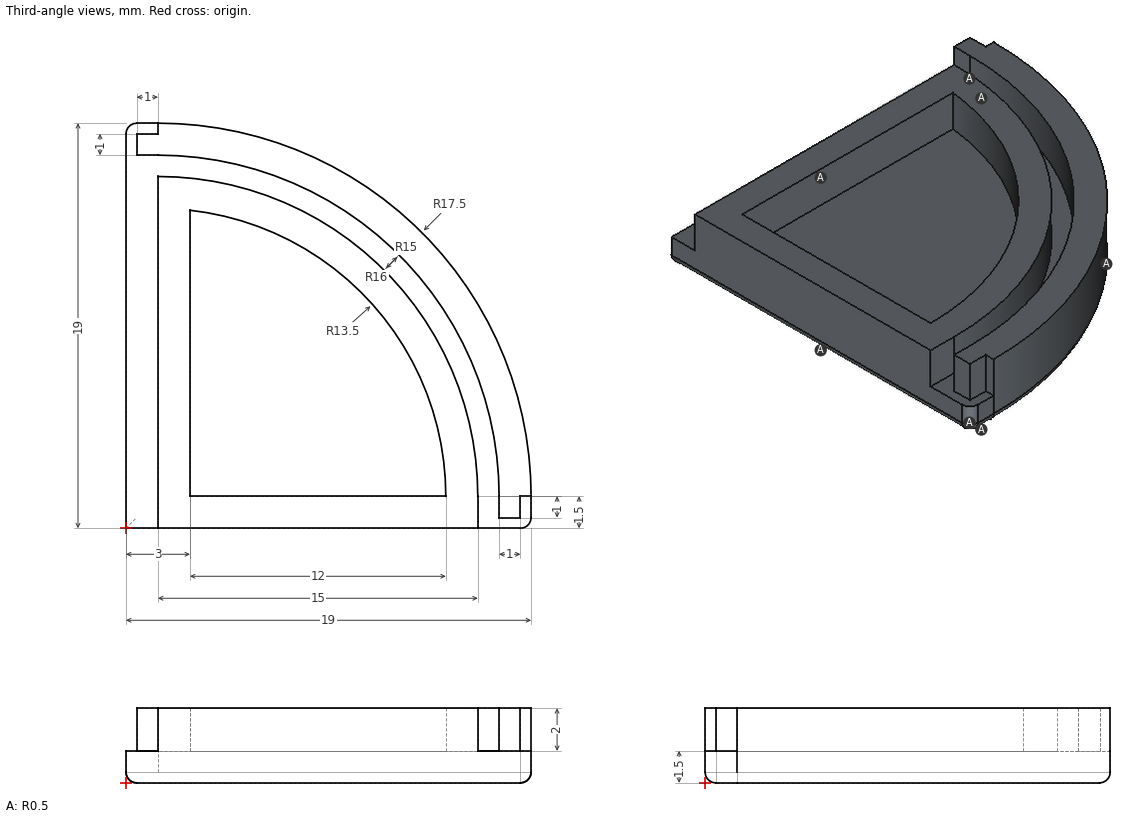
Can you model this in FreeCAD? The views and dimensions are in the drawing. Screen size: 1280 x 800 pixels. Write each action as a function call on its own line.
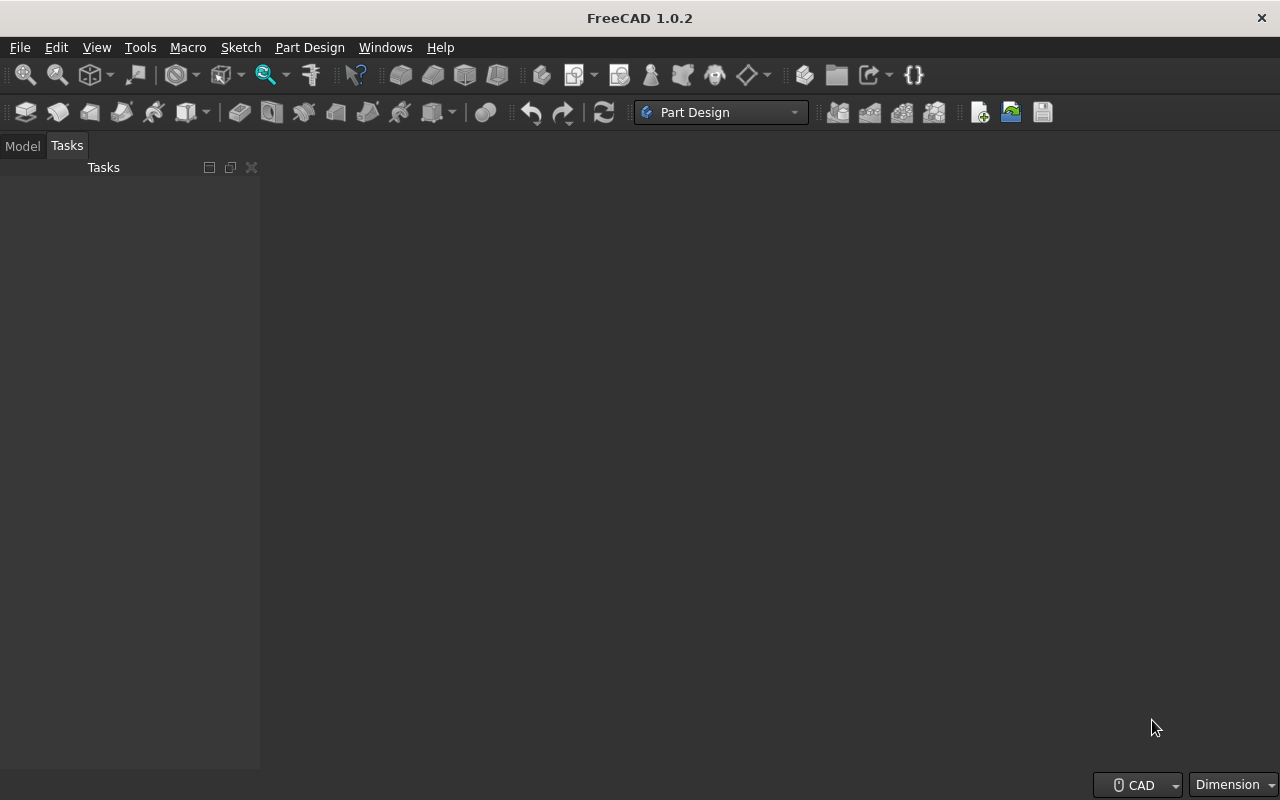
key(ctrl+n)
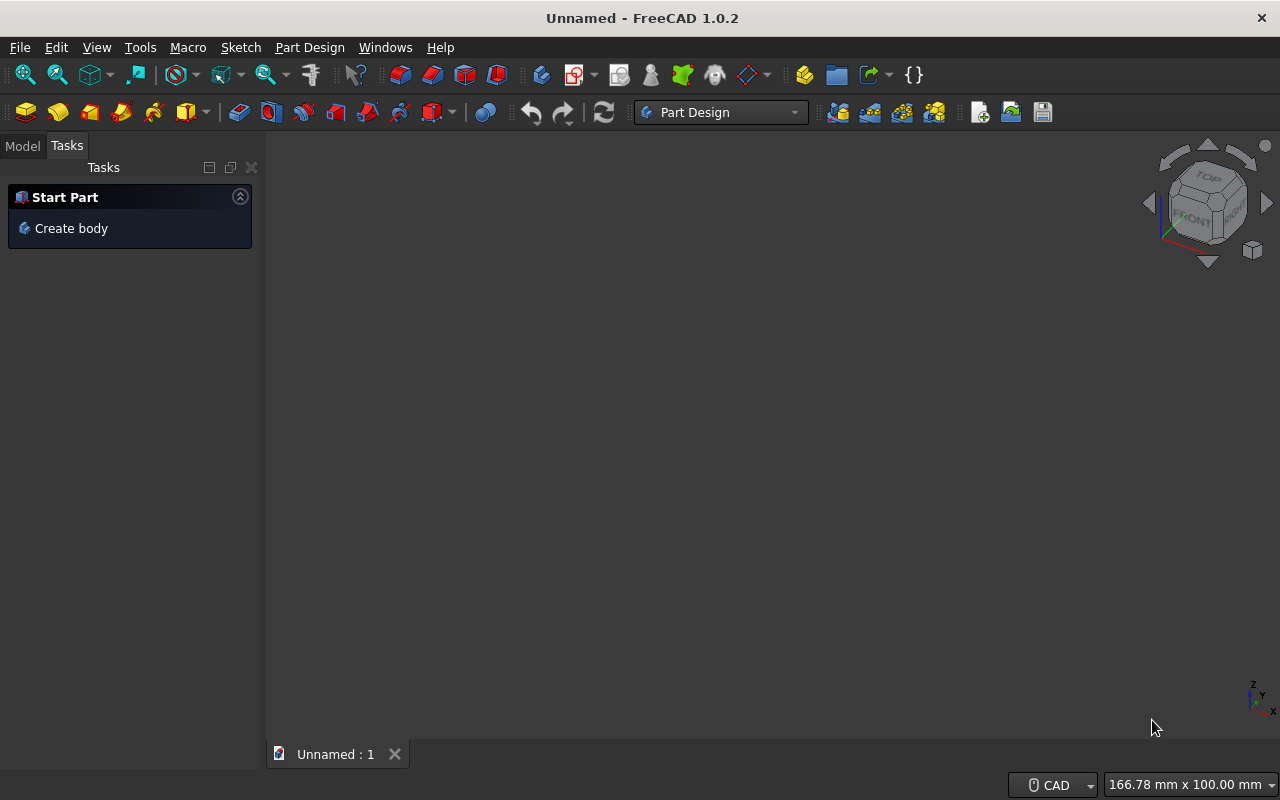
click(574, 76)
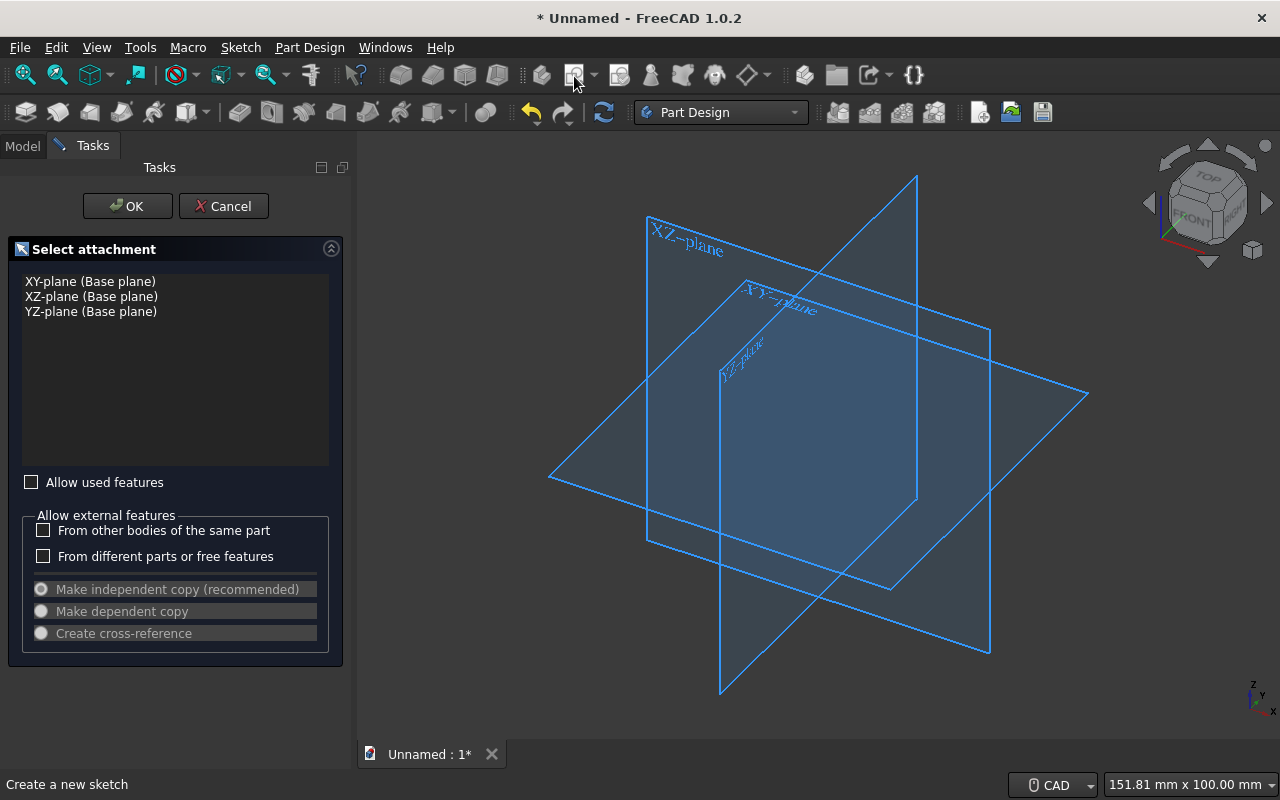
click(82, 282)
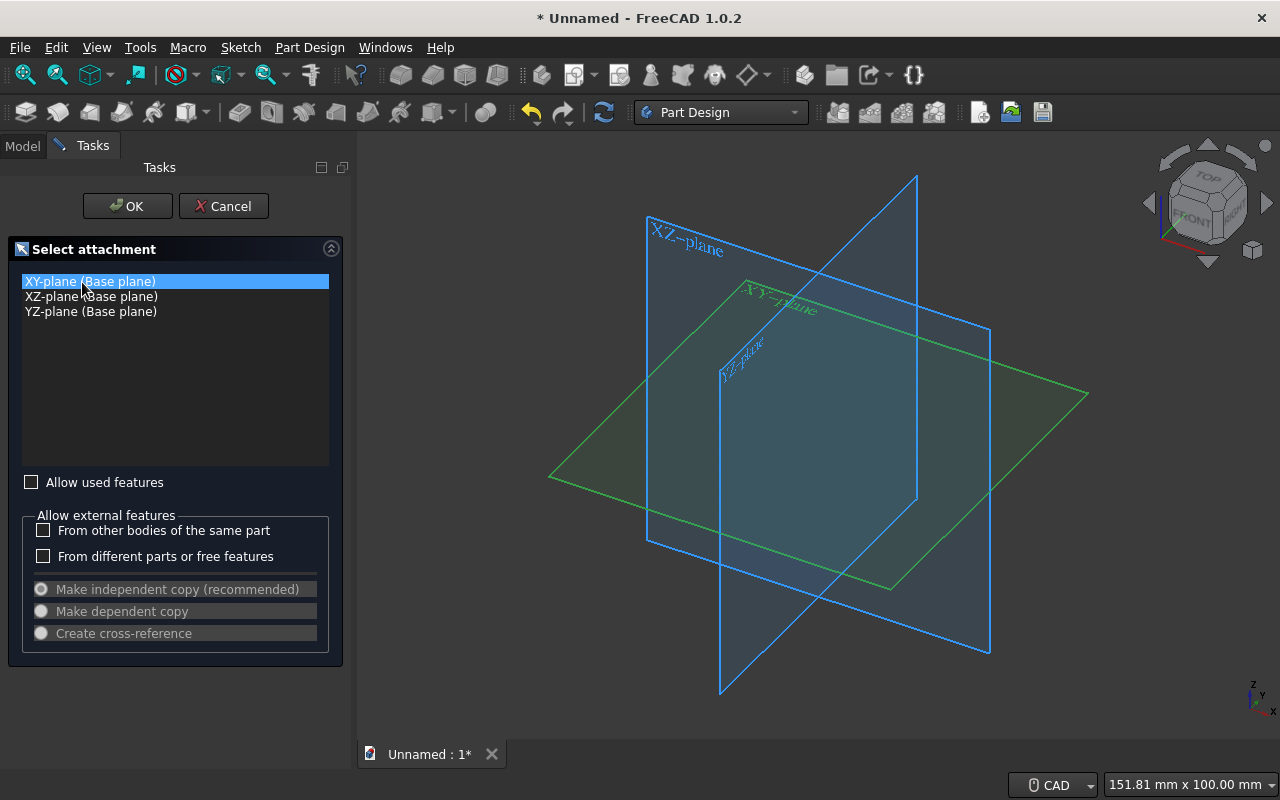
click(128, 206)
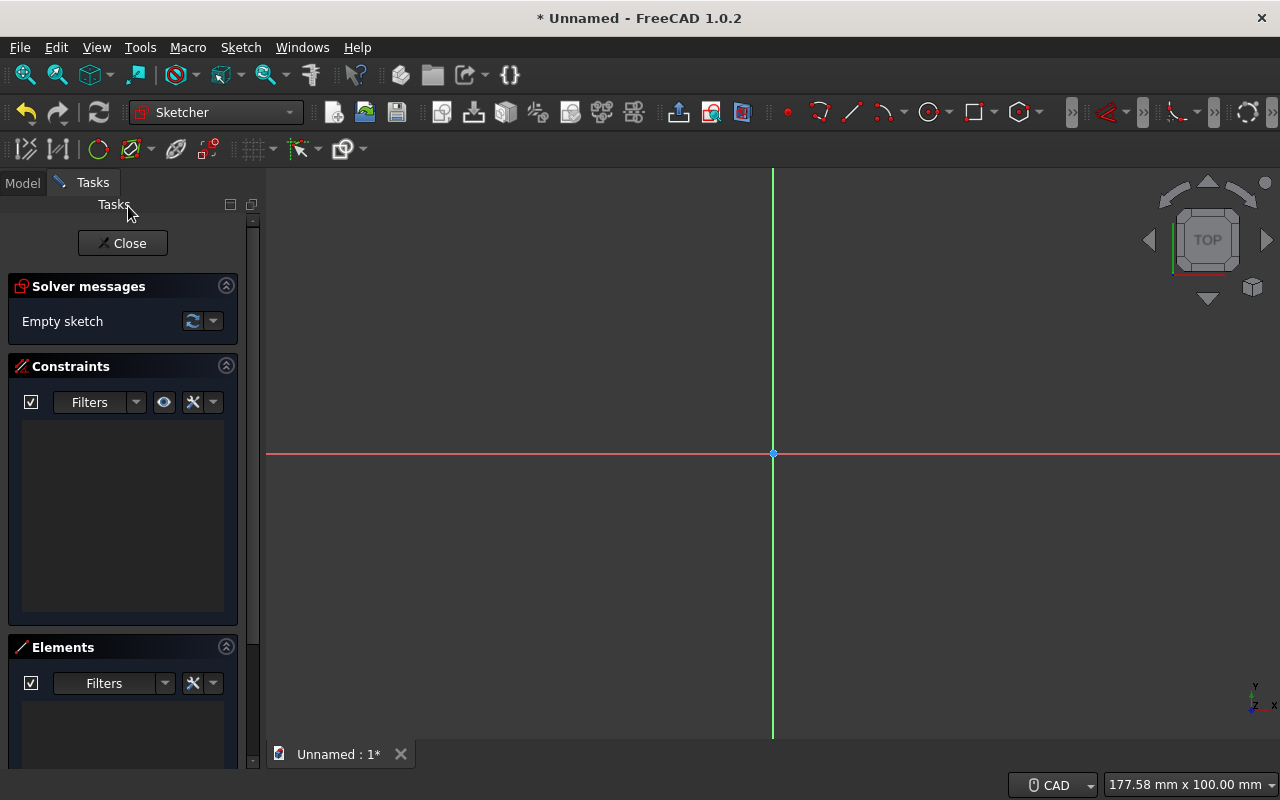
scroll(880, 376, up, 6)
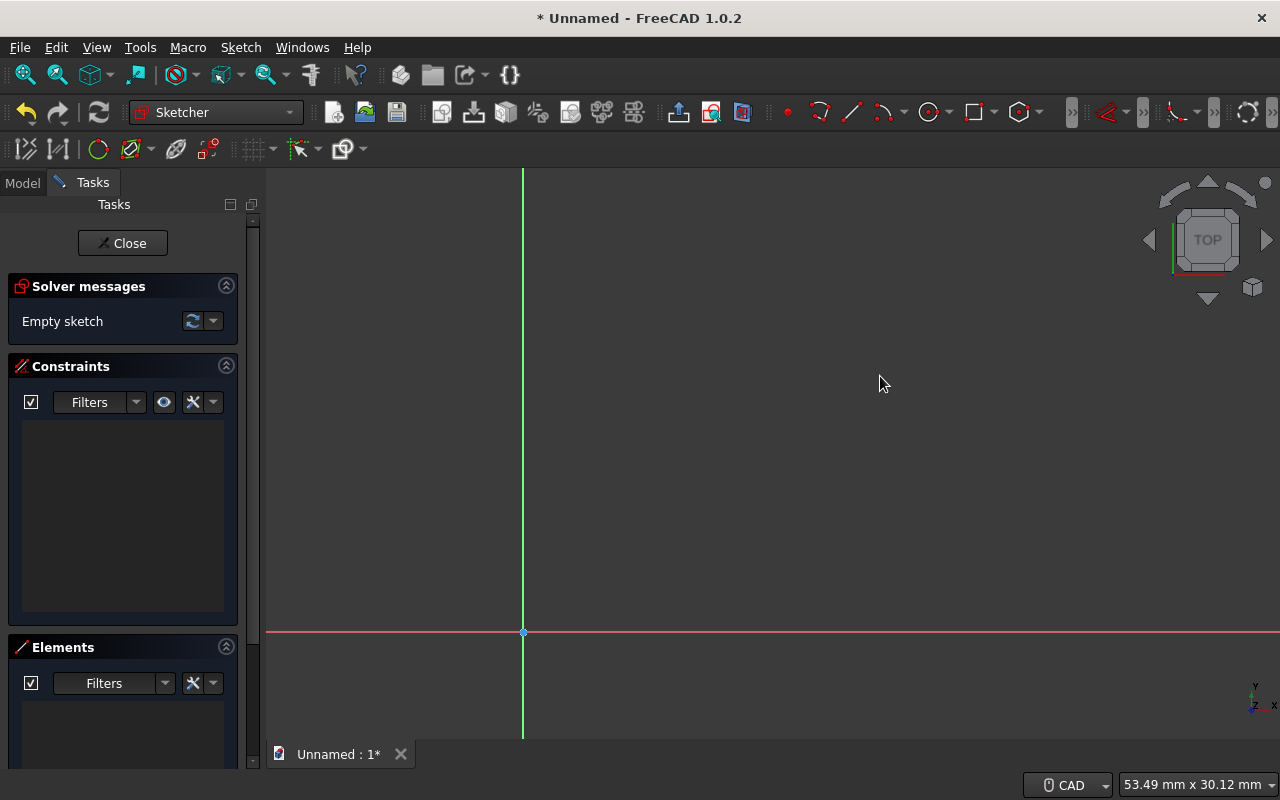
click(820, 112)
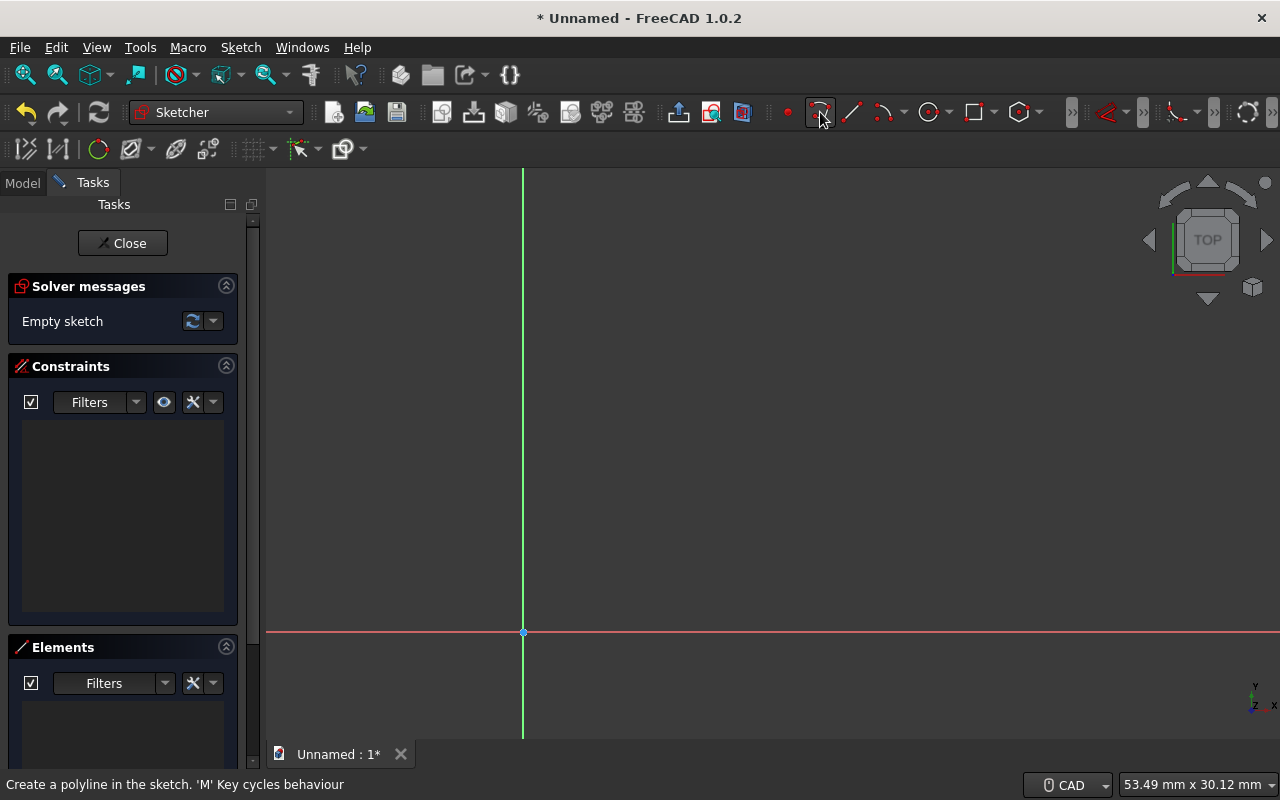
click(552, 272)
click(523, 272)
click(523, 632)
click(884, 623)
click(884, 604)
right_click(884, 604)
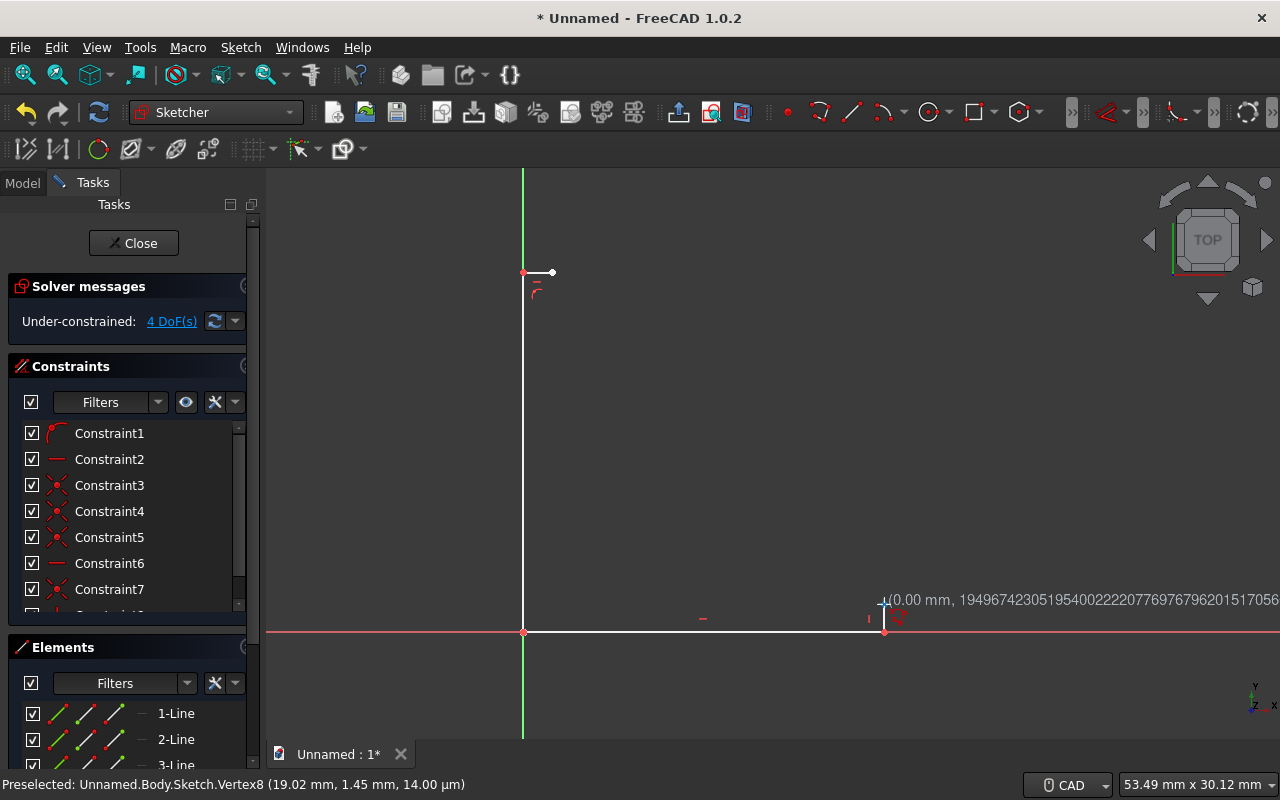
key(g)
key(3)
key(a)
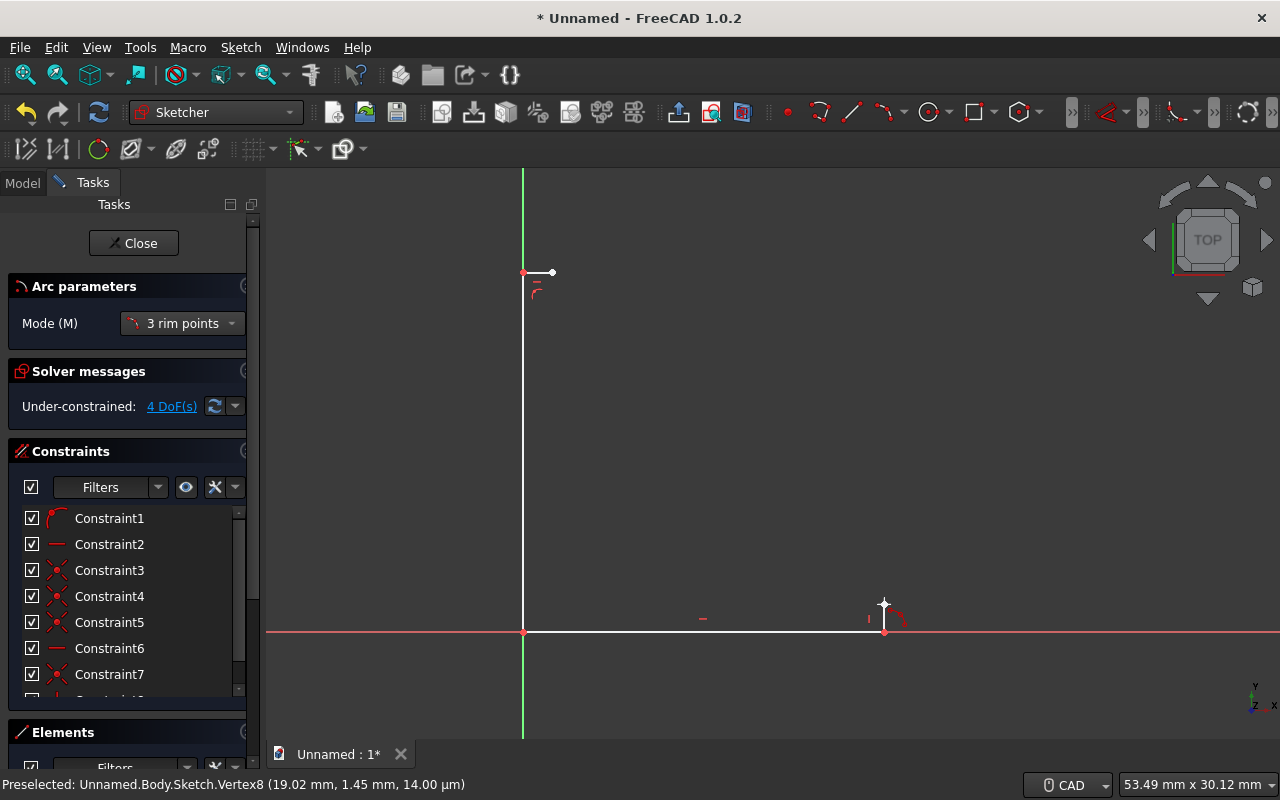
click(884, 605)
click(552, 273)
click(786, 369)
key(Escape)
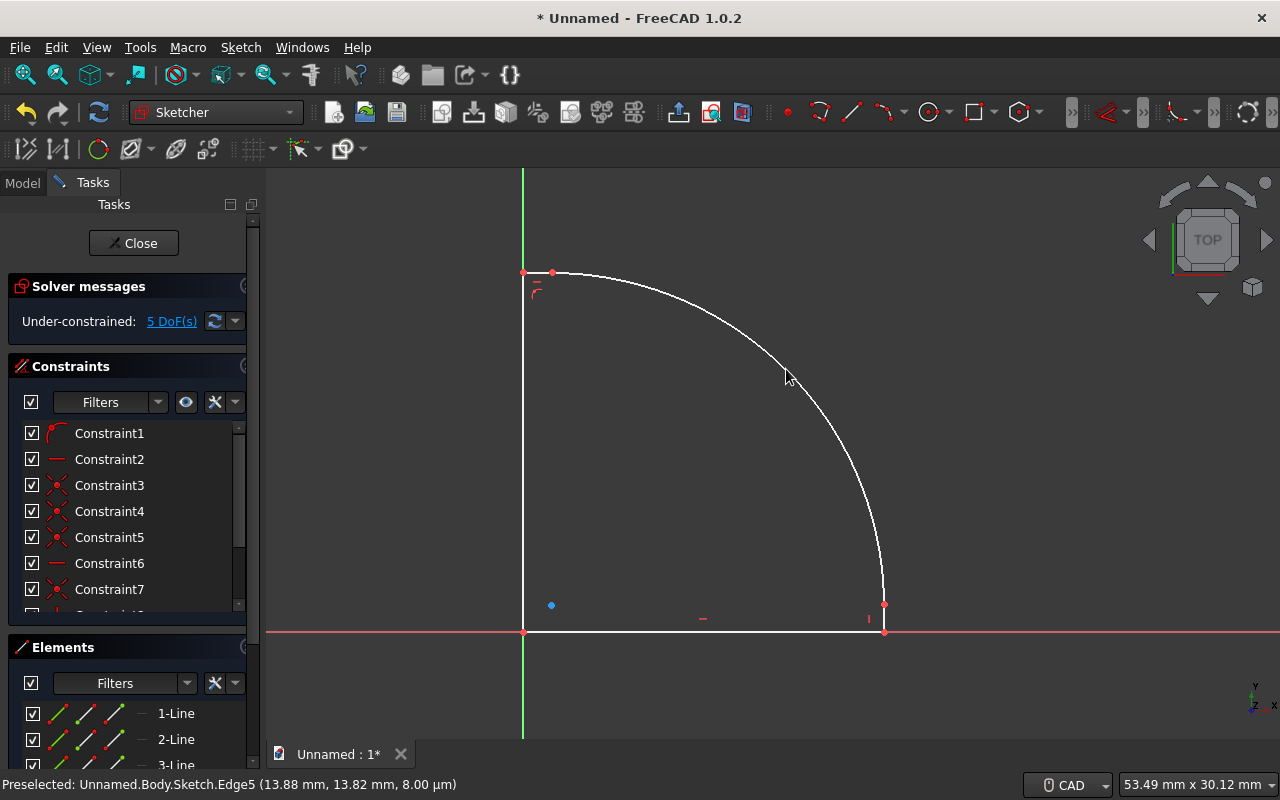
click(541, 273)